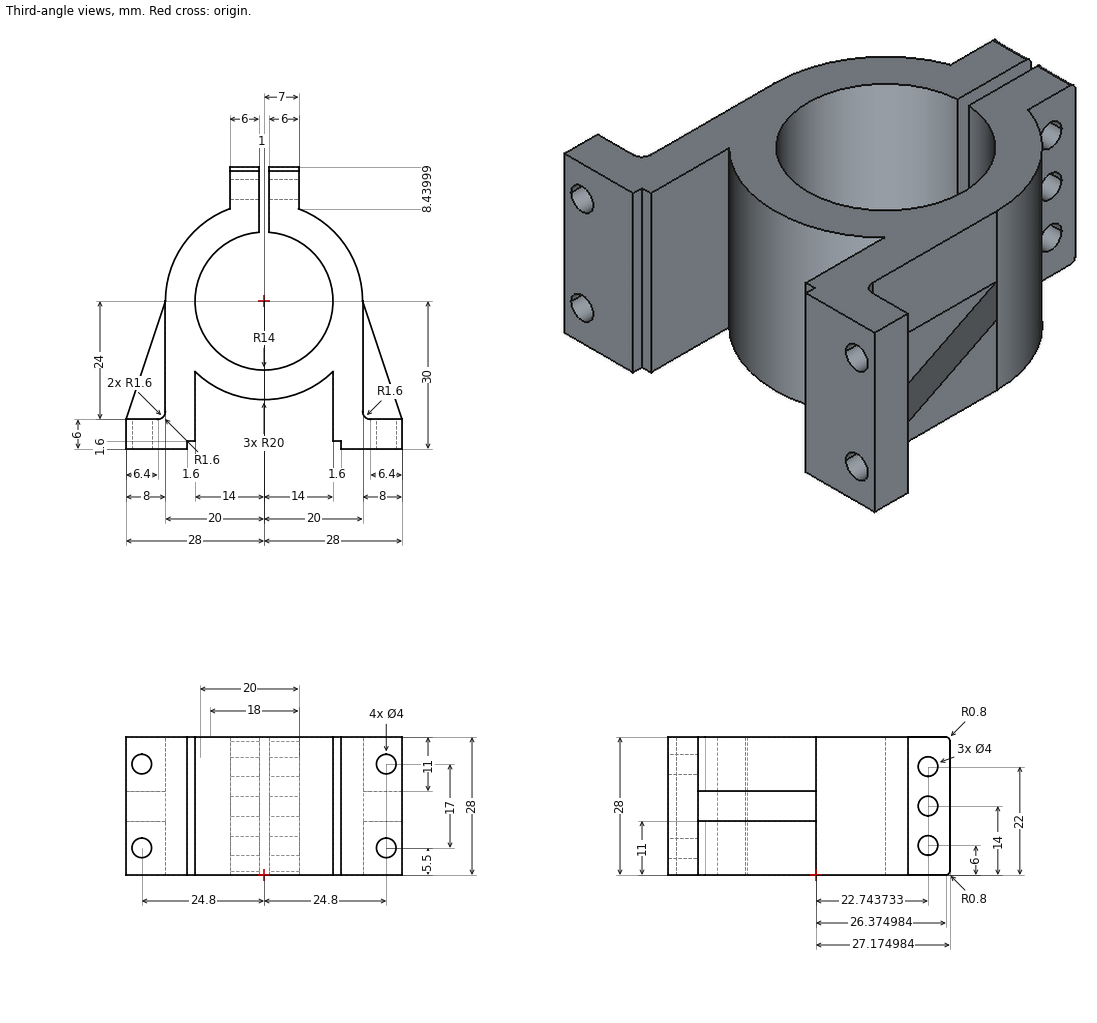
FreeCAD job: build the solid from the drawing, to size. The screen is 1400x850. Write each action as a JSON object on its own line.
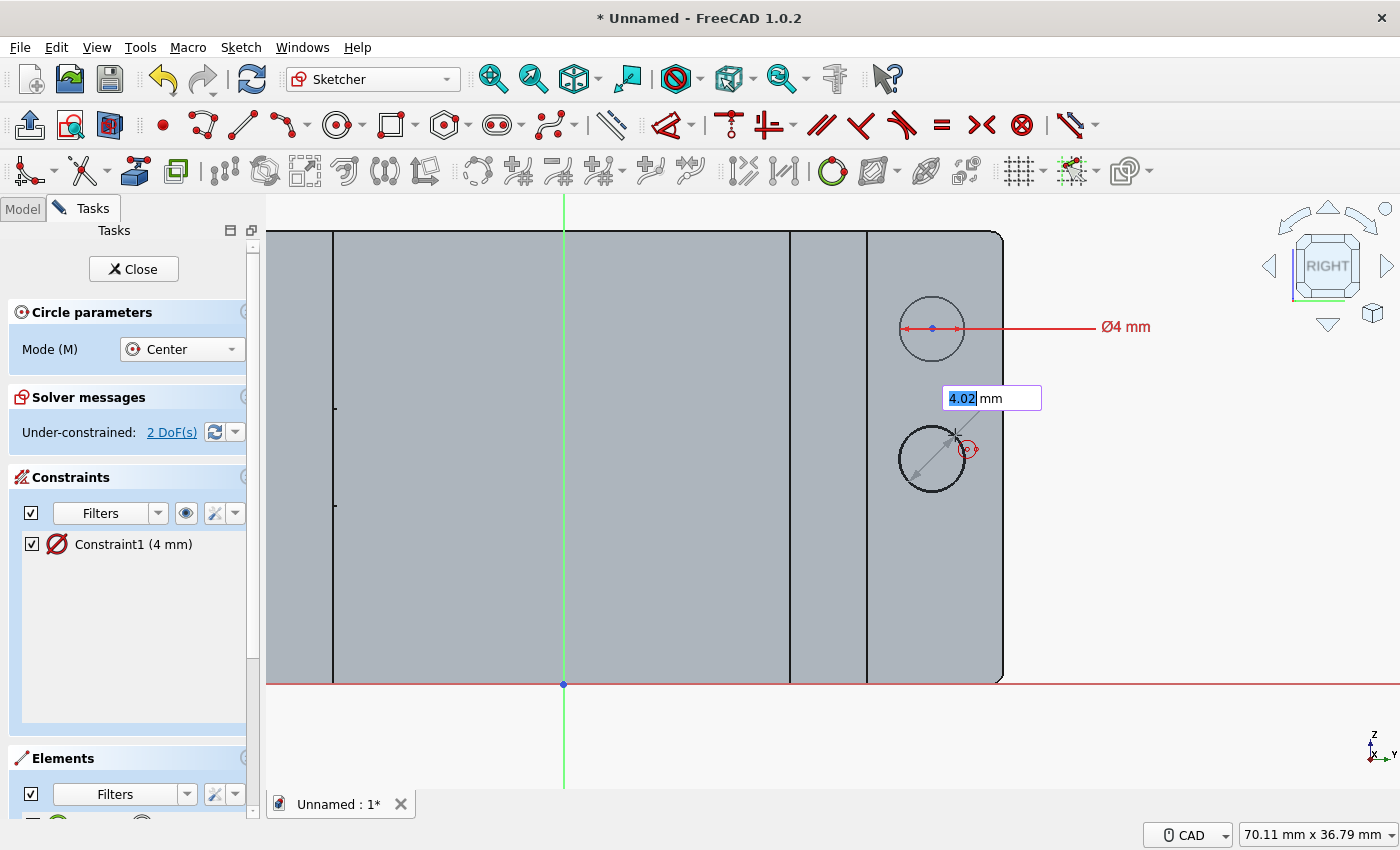
{"action": "type", "text": "4"}
{"action": "key", "text": "Return"}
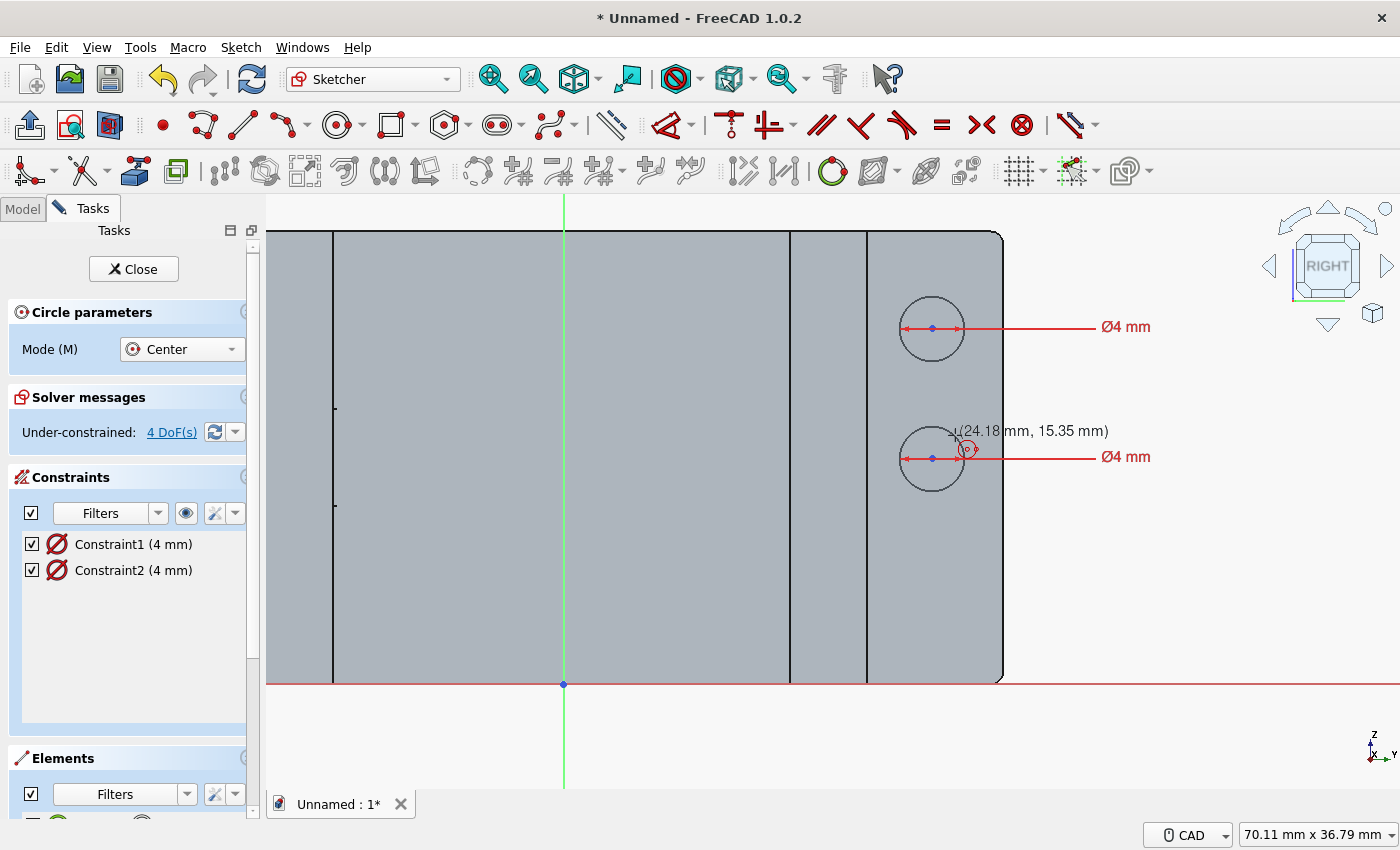
{"action": "left_click", "coordinate": [932, 587]}
{"action": "mouse_move", "coordinate": [955, 564]}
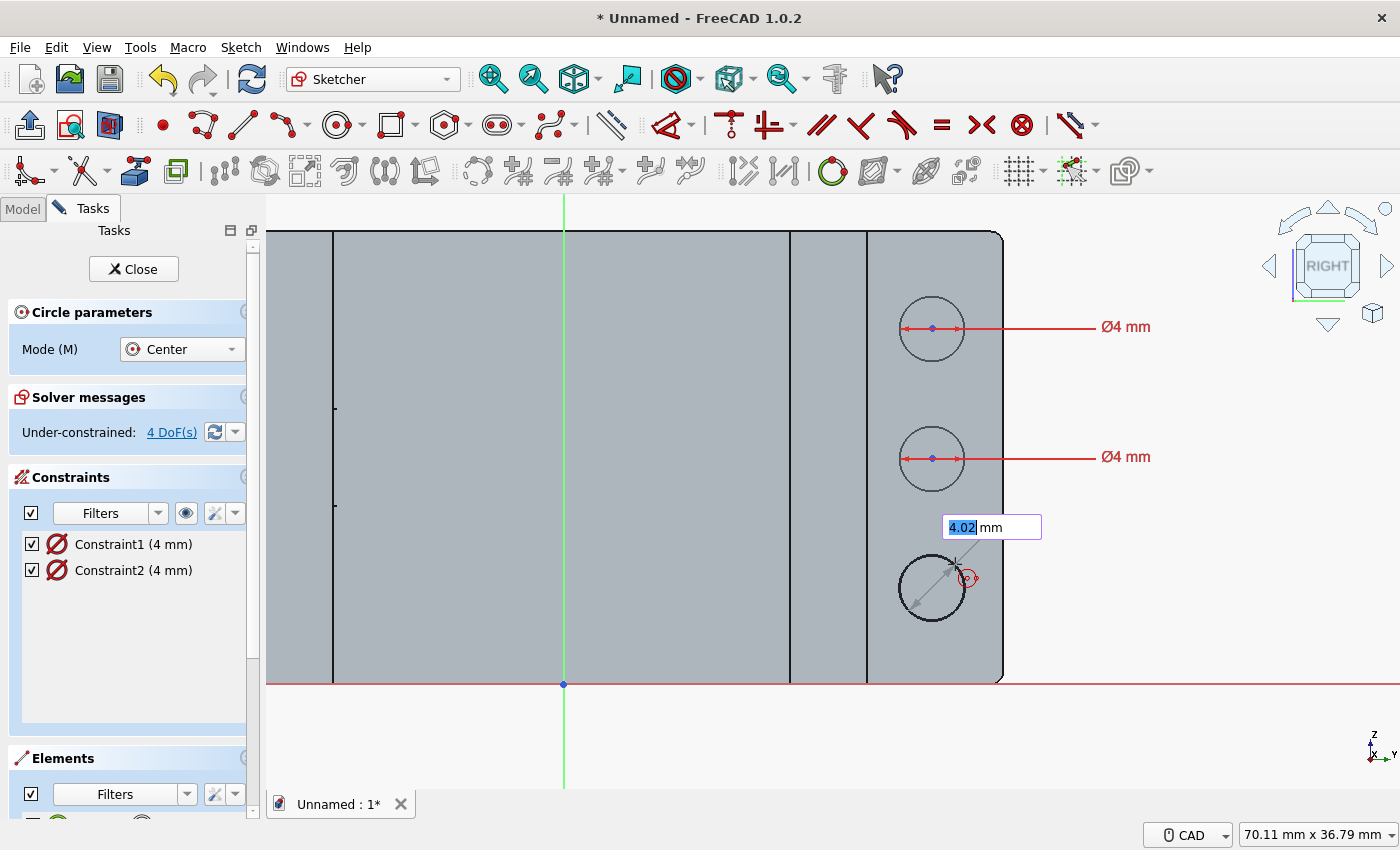
{"action": "type", "text": "4"}
{"action": "key", "text": "Return"}
{"action": "key", "text": "Escape"}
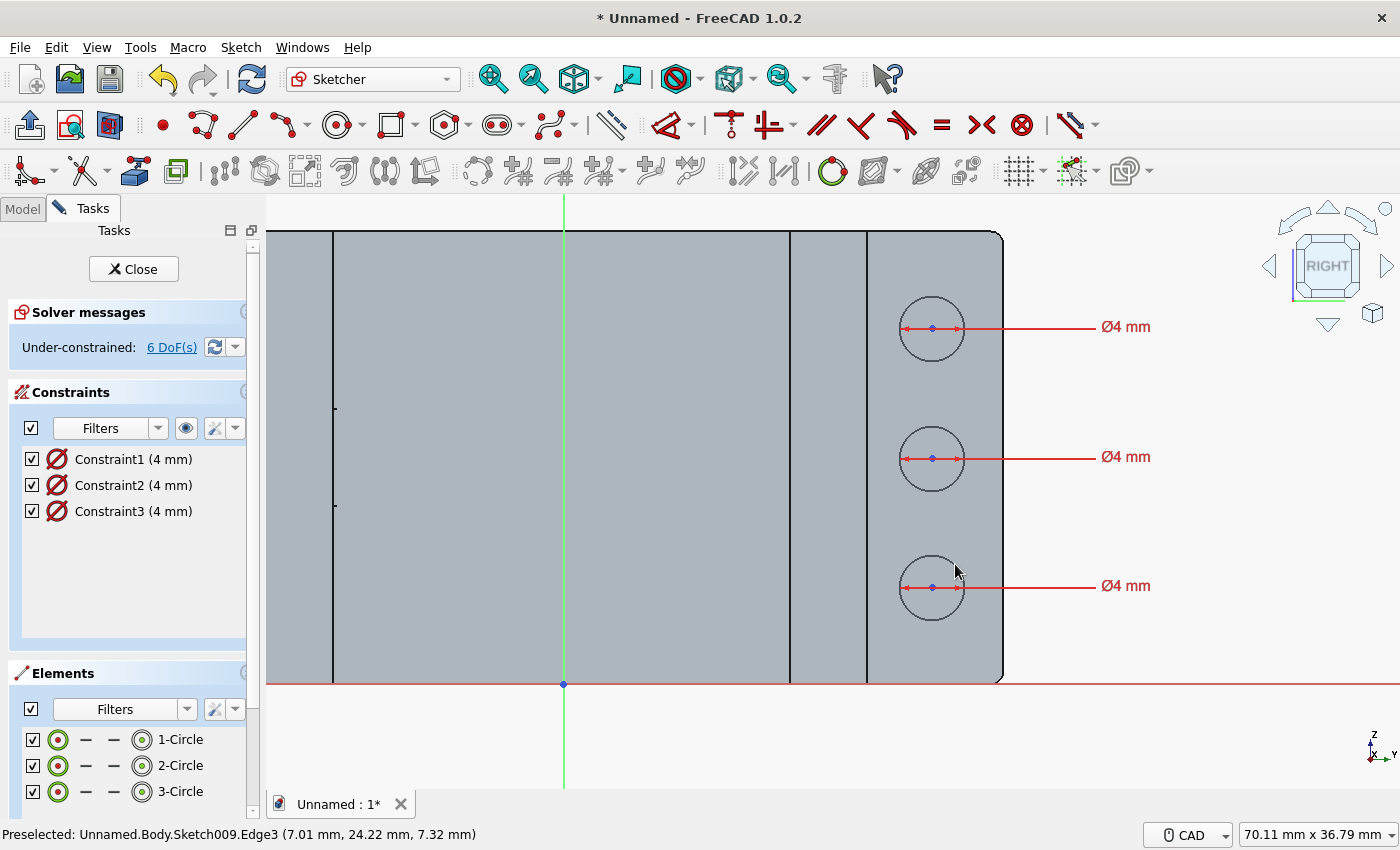
{"action": "left_click", "coordinate": [932, 329]}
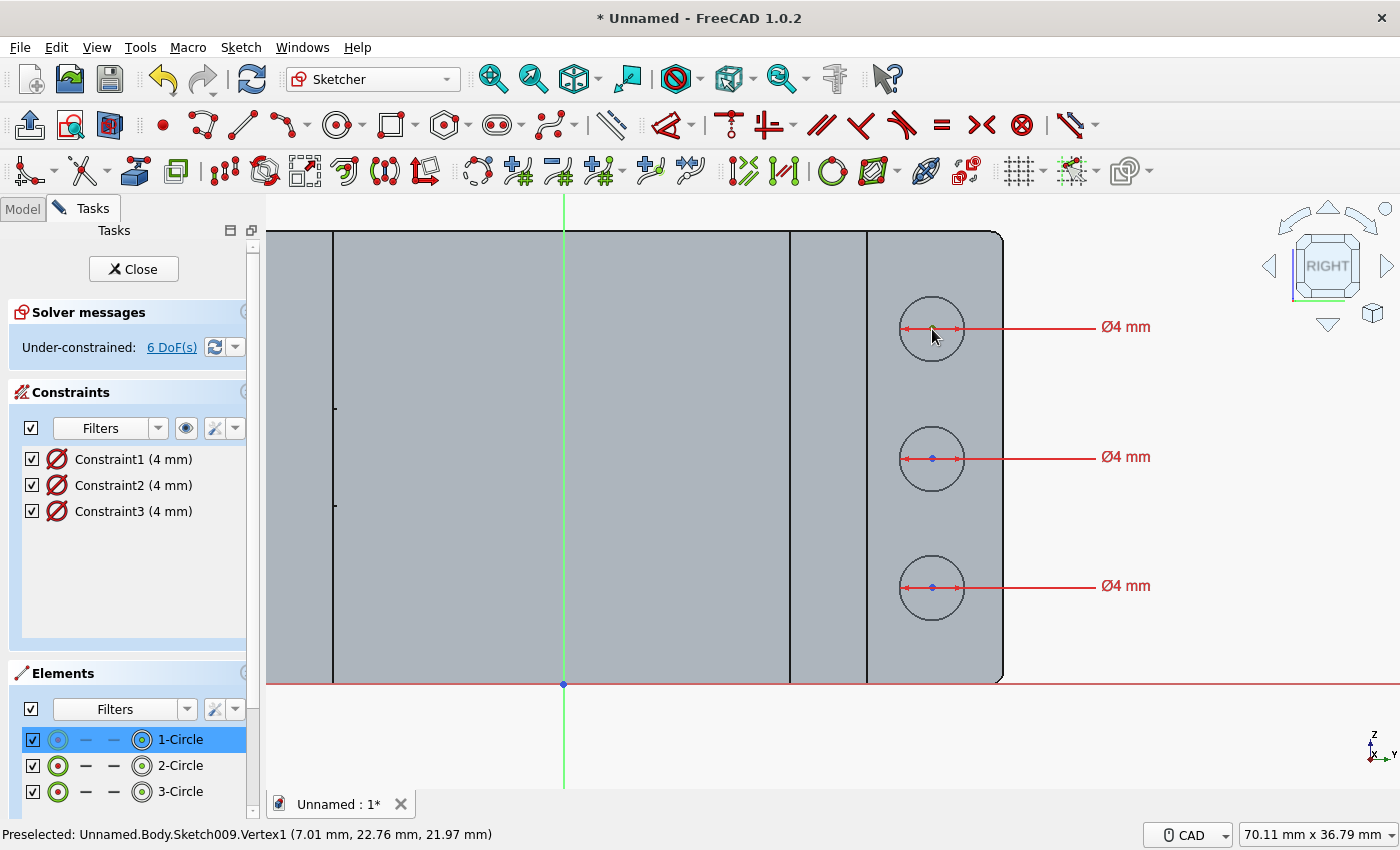
{"action": "left_click", "coordinate": [932, 459]}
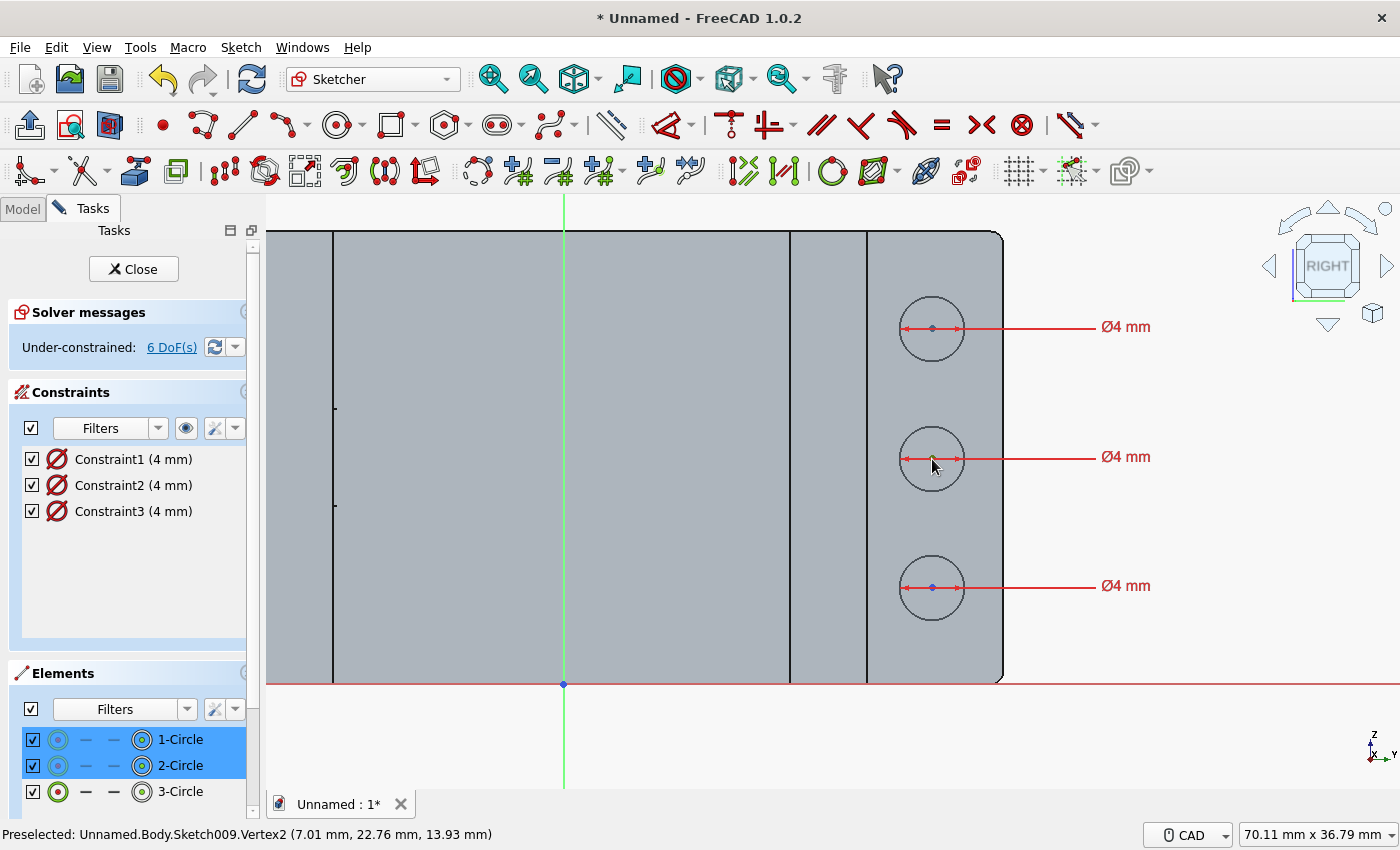
{"action": "left_click", "coordinate": [796, 126]}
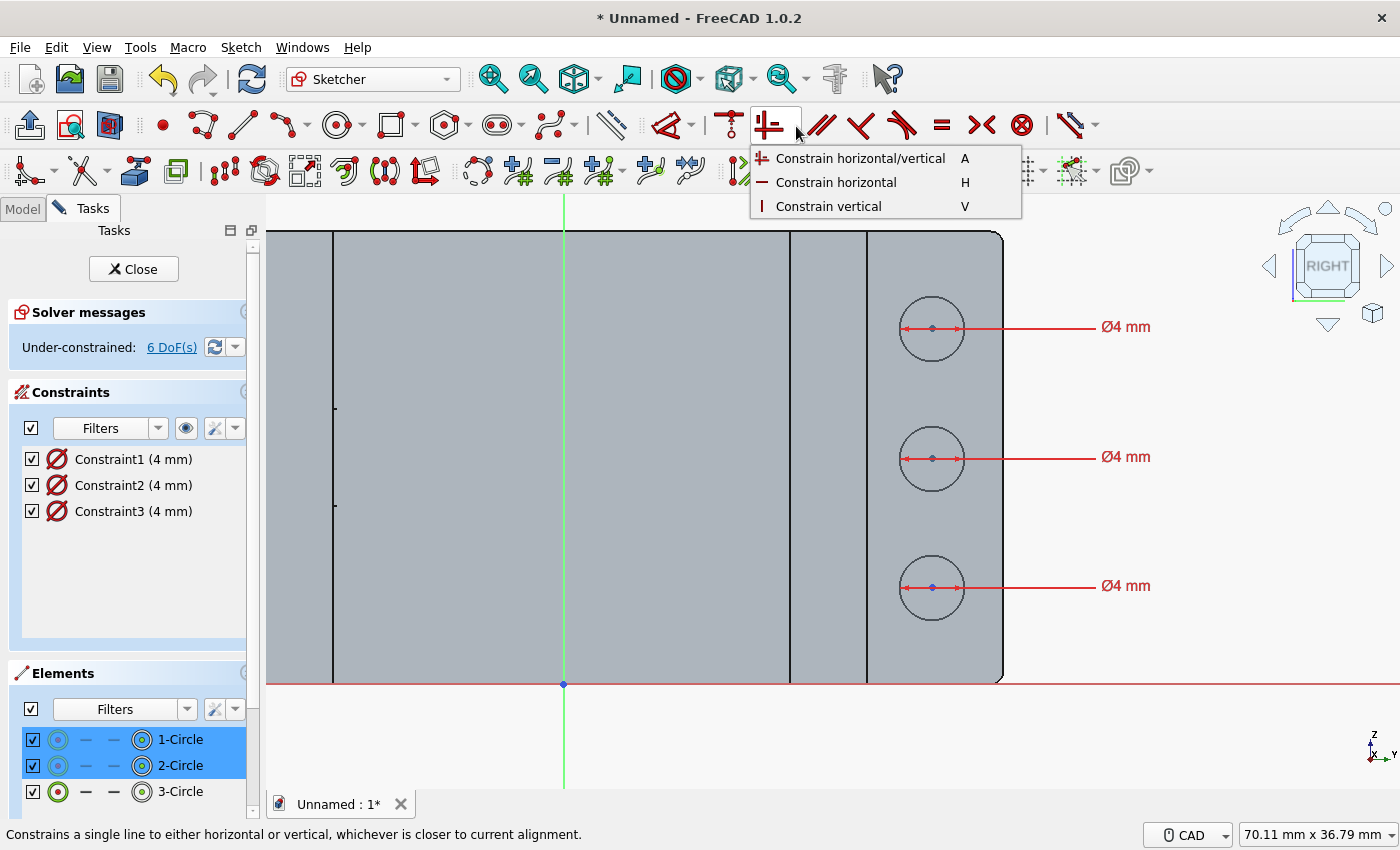
{"action": "left_click", "coordinate": [886, 206]}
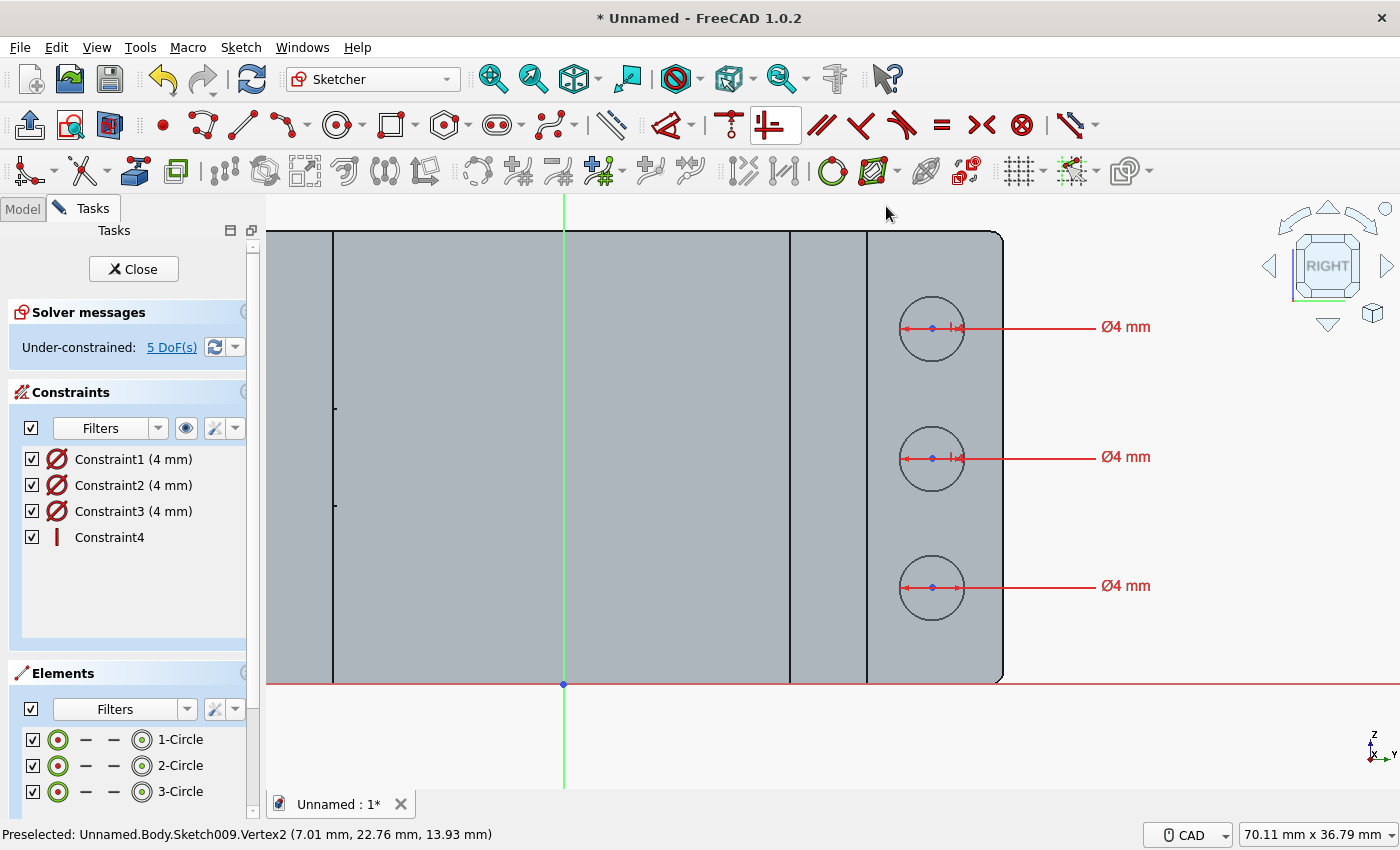
{"action": "left_click", "coordinate": [932, 459]}